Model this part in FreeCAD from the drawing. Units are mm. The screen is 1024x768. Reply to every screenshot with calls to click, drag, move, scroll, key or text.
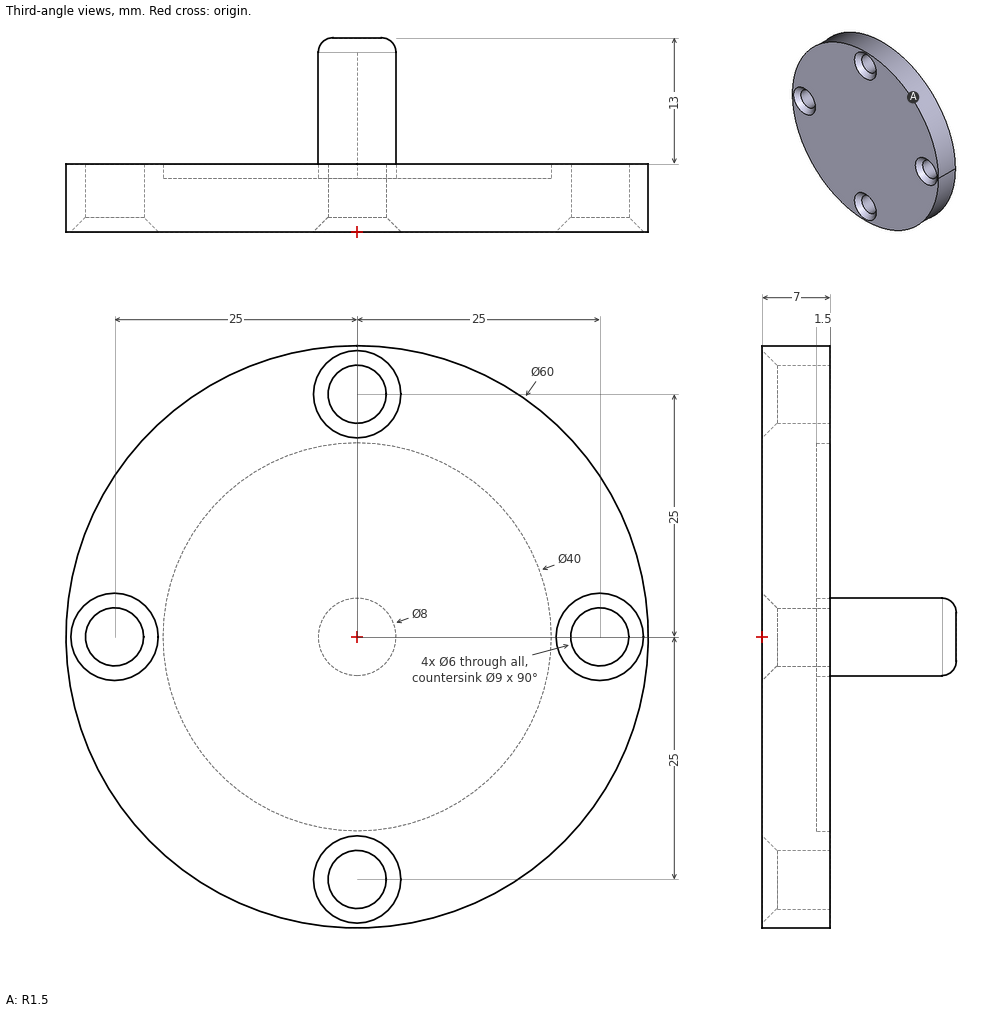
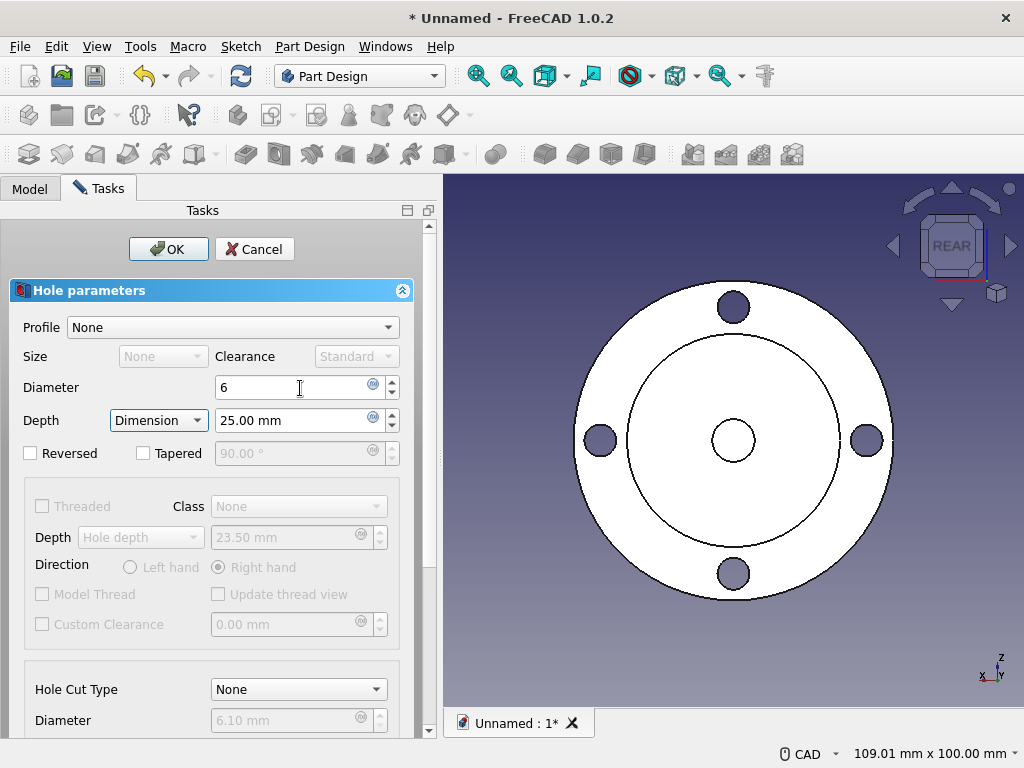
click(160, 420)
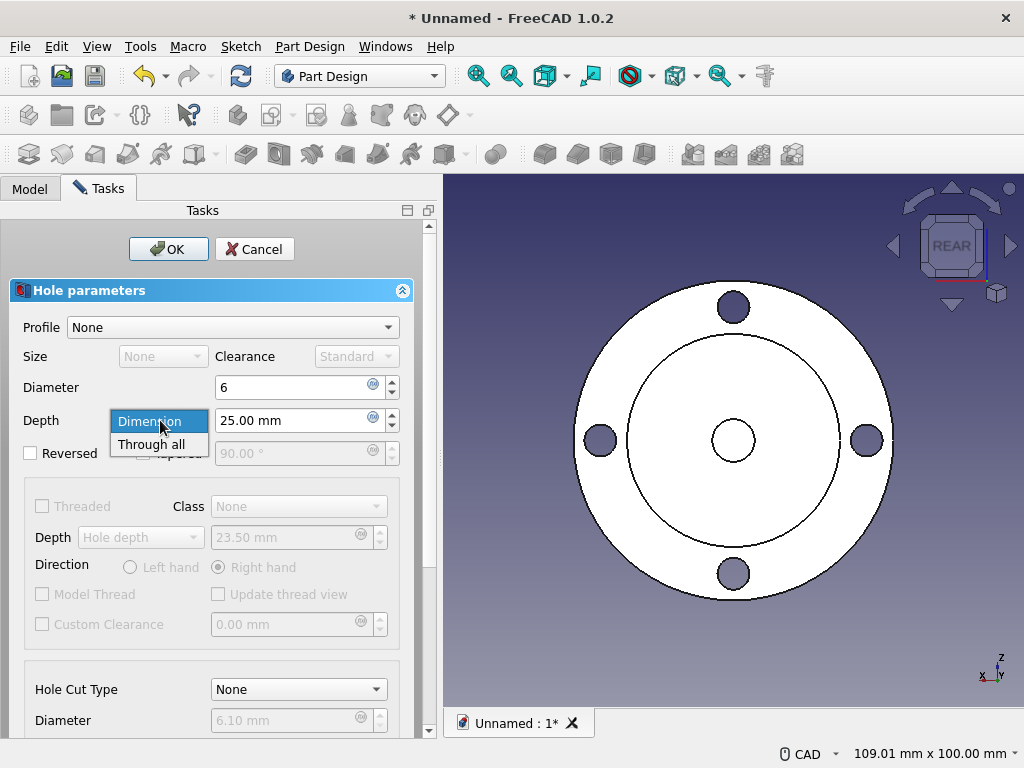
click(158, 444)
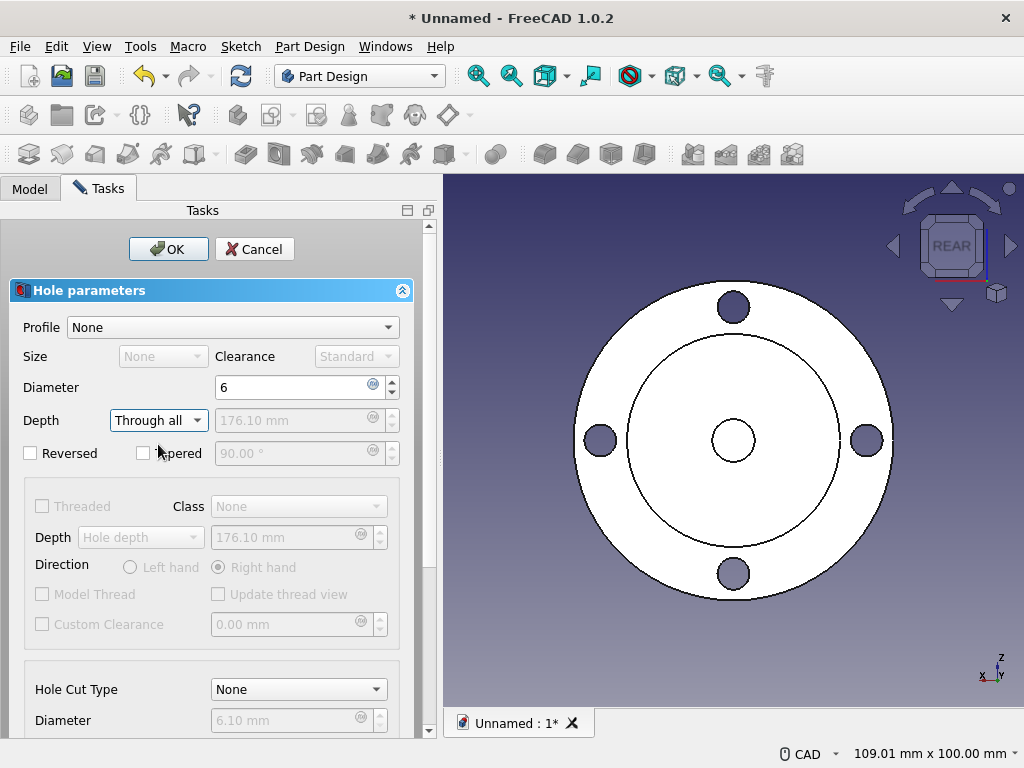
click(300, 690)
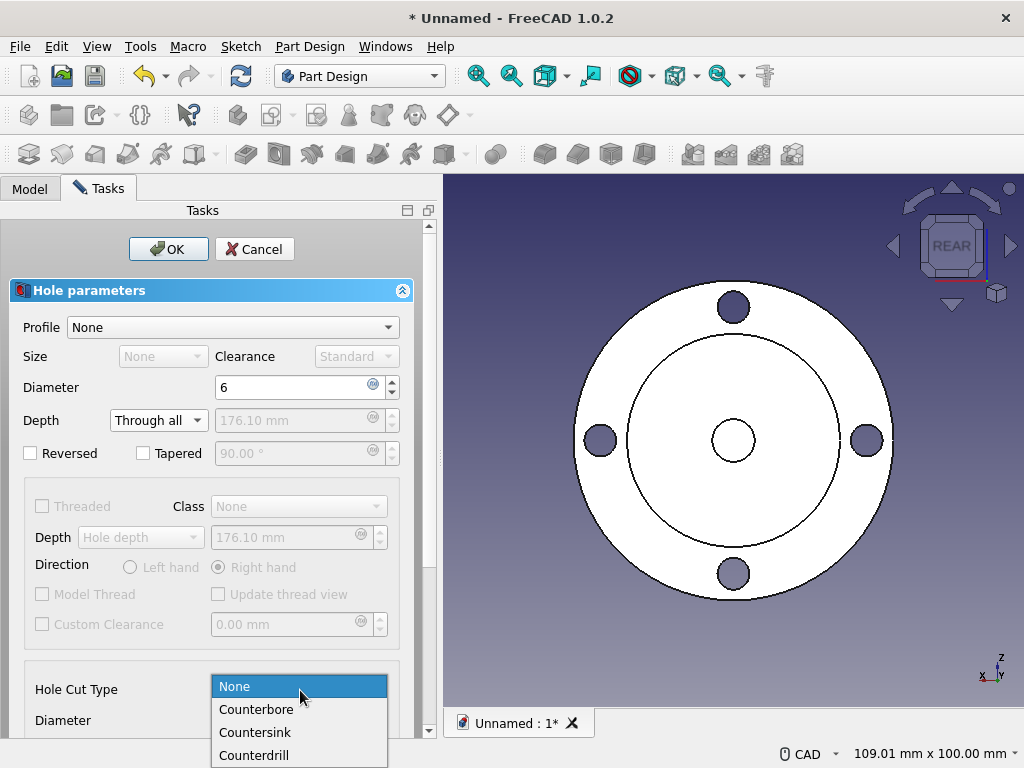
click(298, 732)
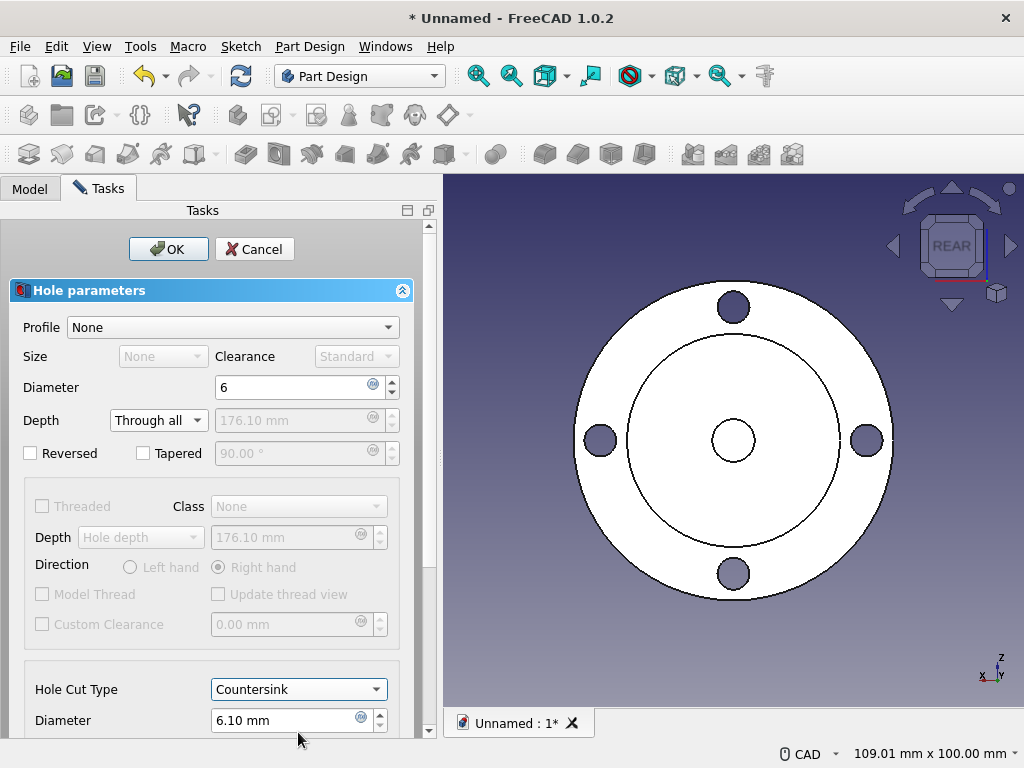
triple_click(292, 720)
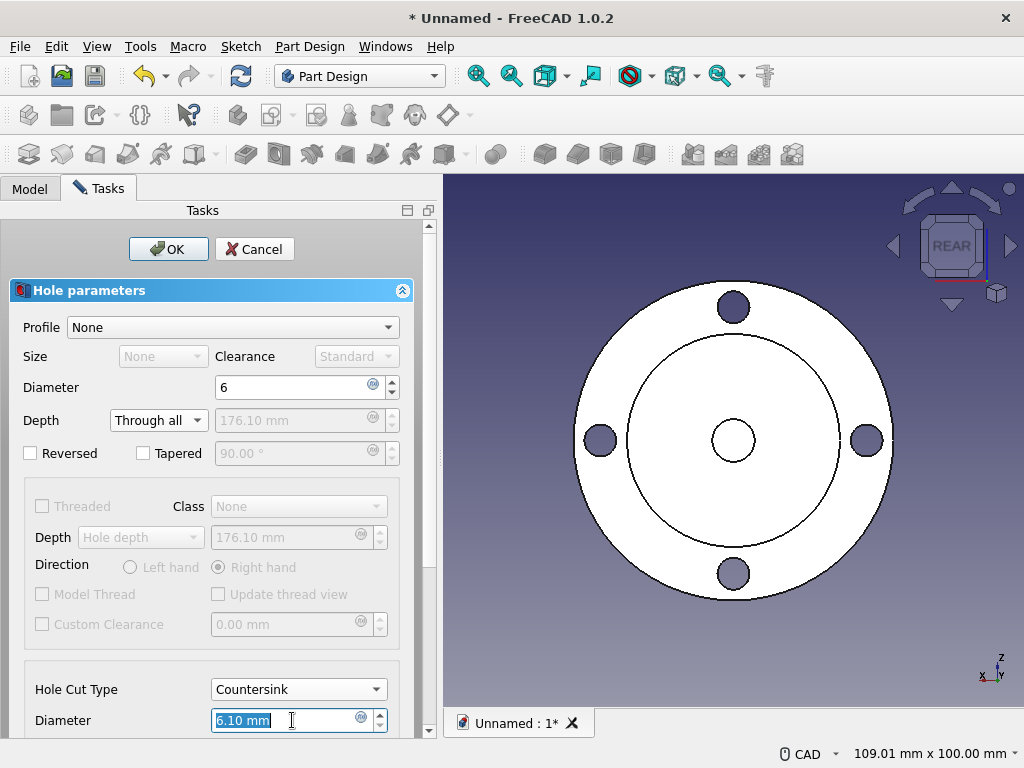
text(9)
key(Tab)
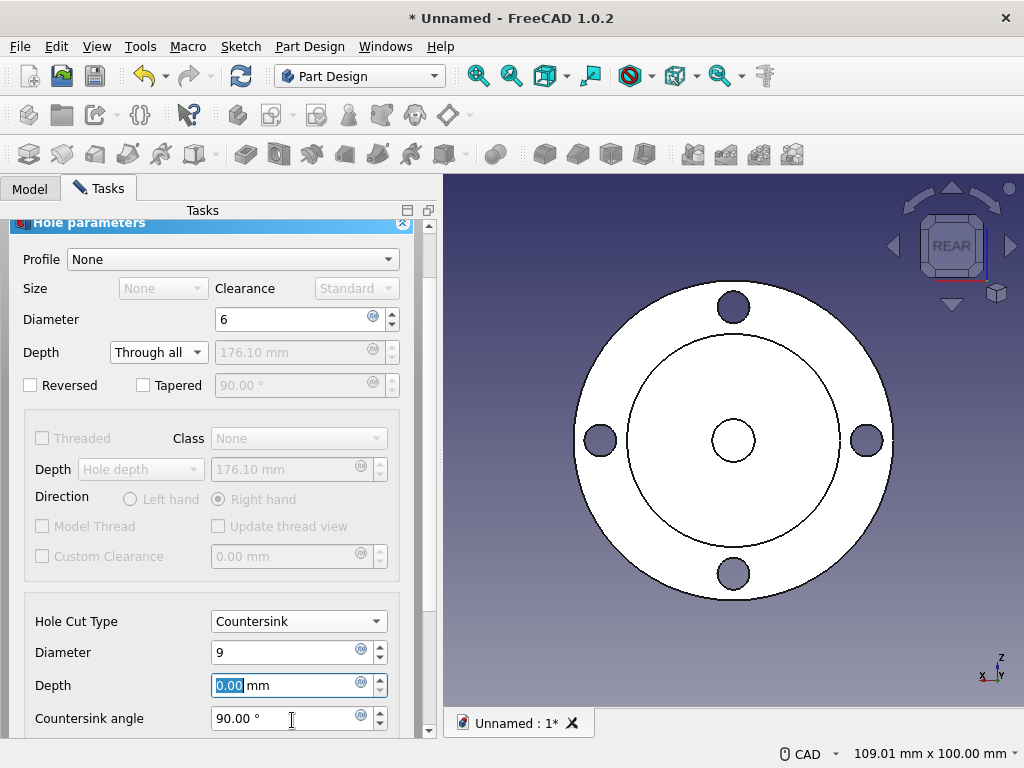
scroll(429, 479, up, 2)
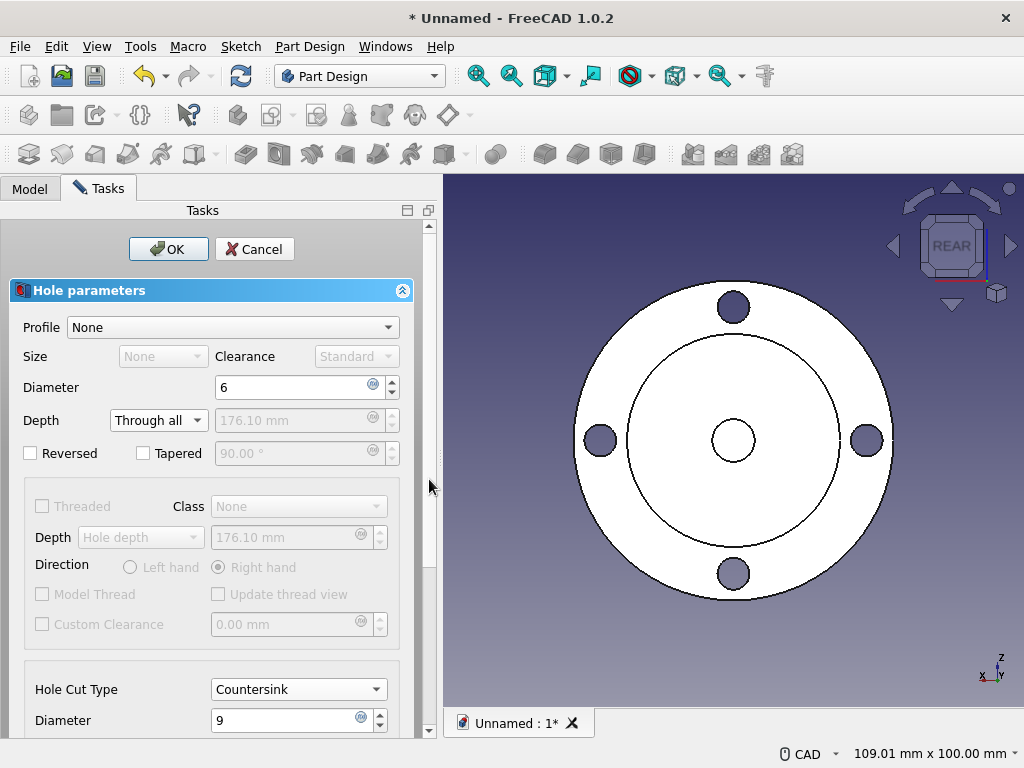
click(169, 249)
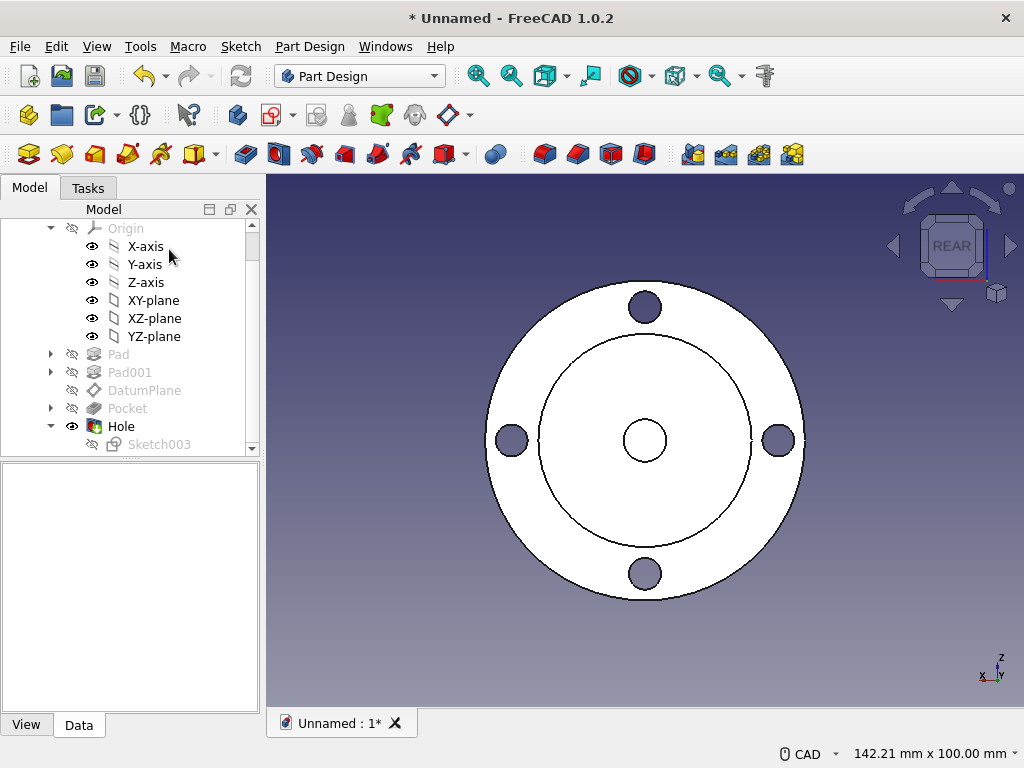
click(666, 439)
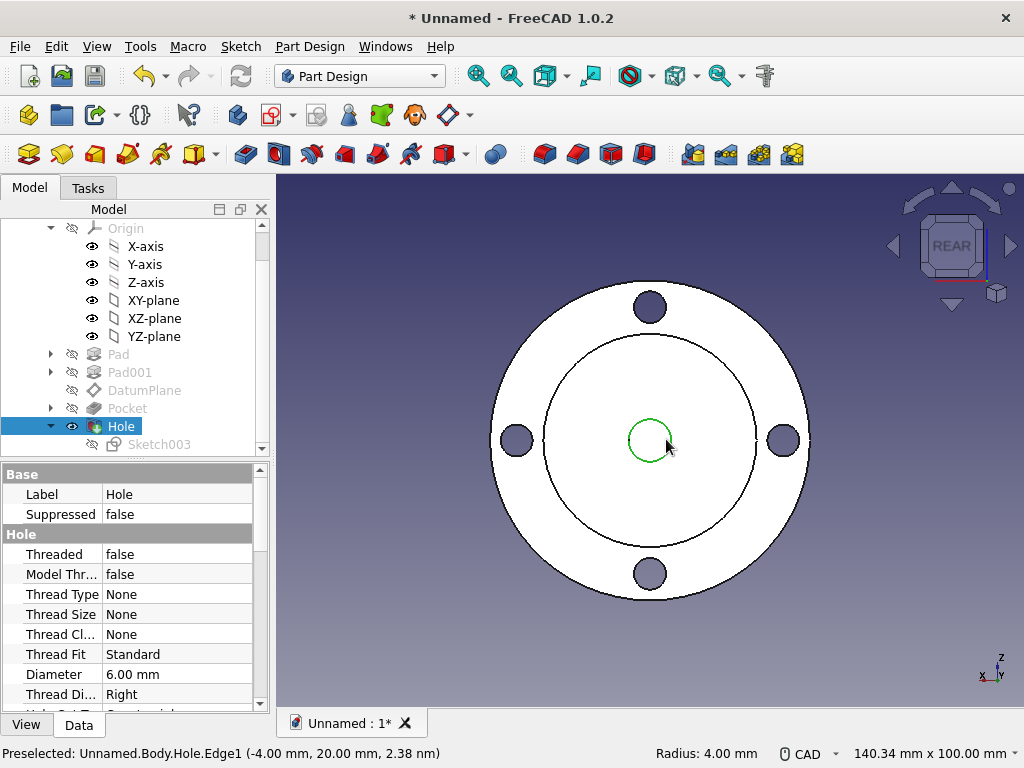
click(545, 154)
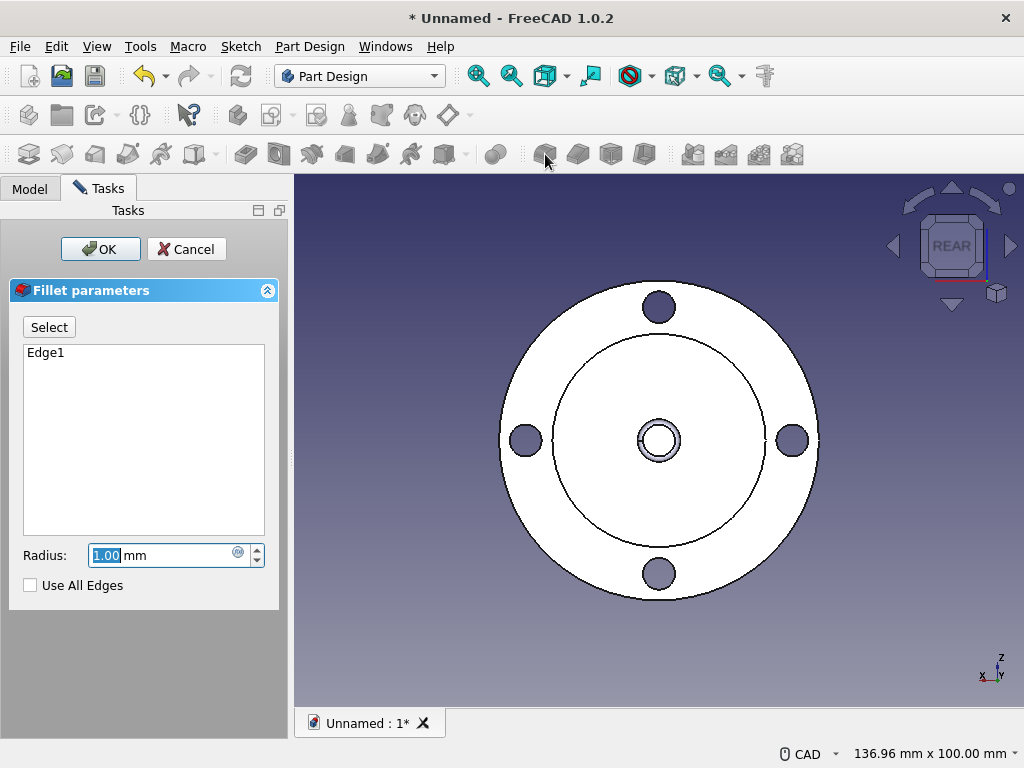
text(1.5)
key(Tab)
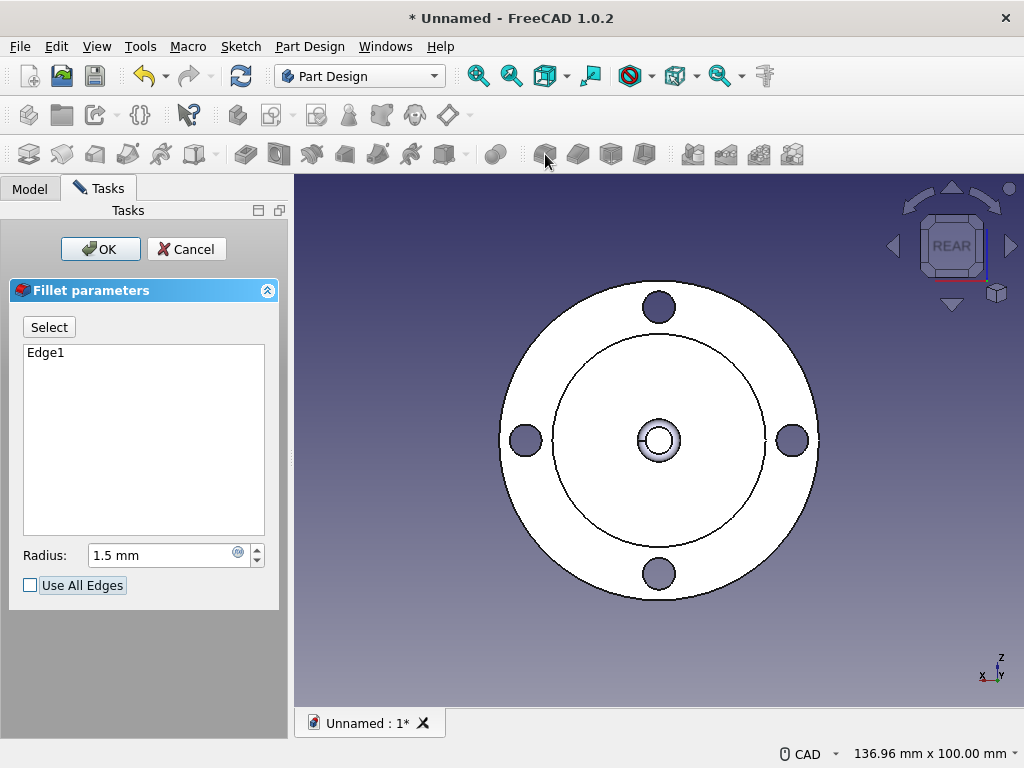
click(101, 249)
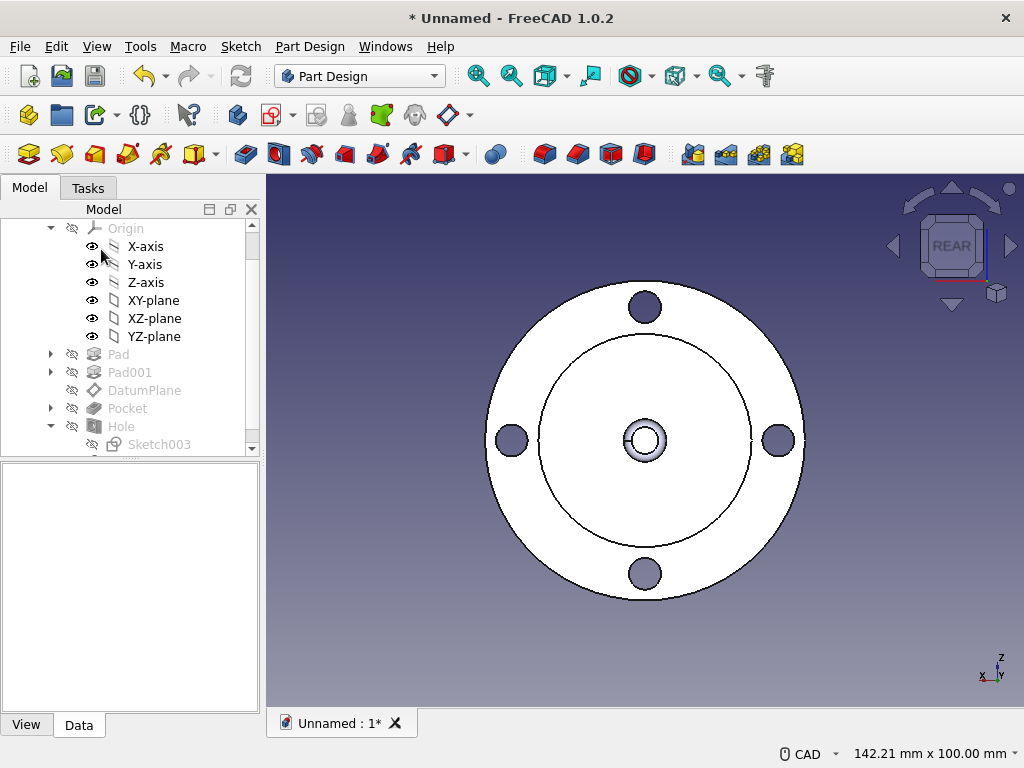
key(0)